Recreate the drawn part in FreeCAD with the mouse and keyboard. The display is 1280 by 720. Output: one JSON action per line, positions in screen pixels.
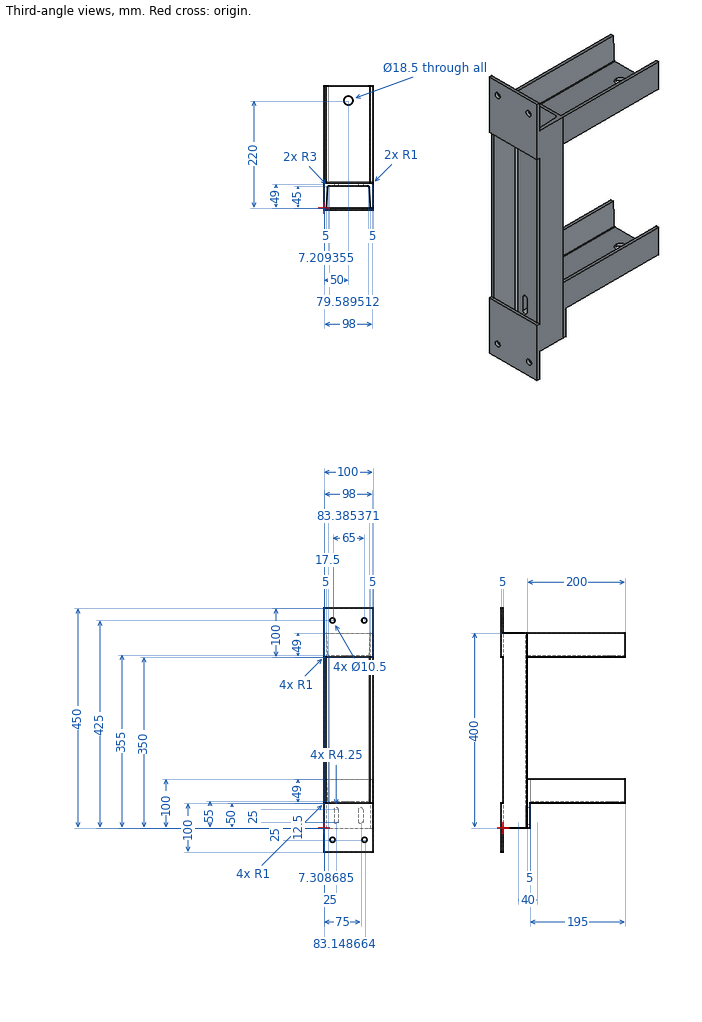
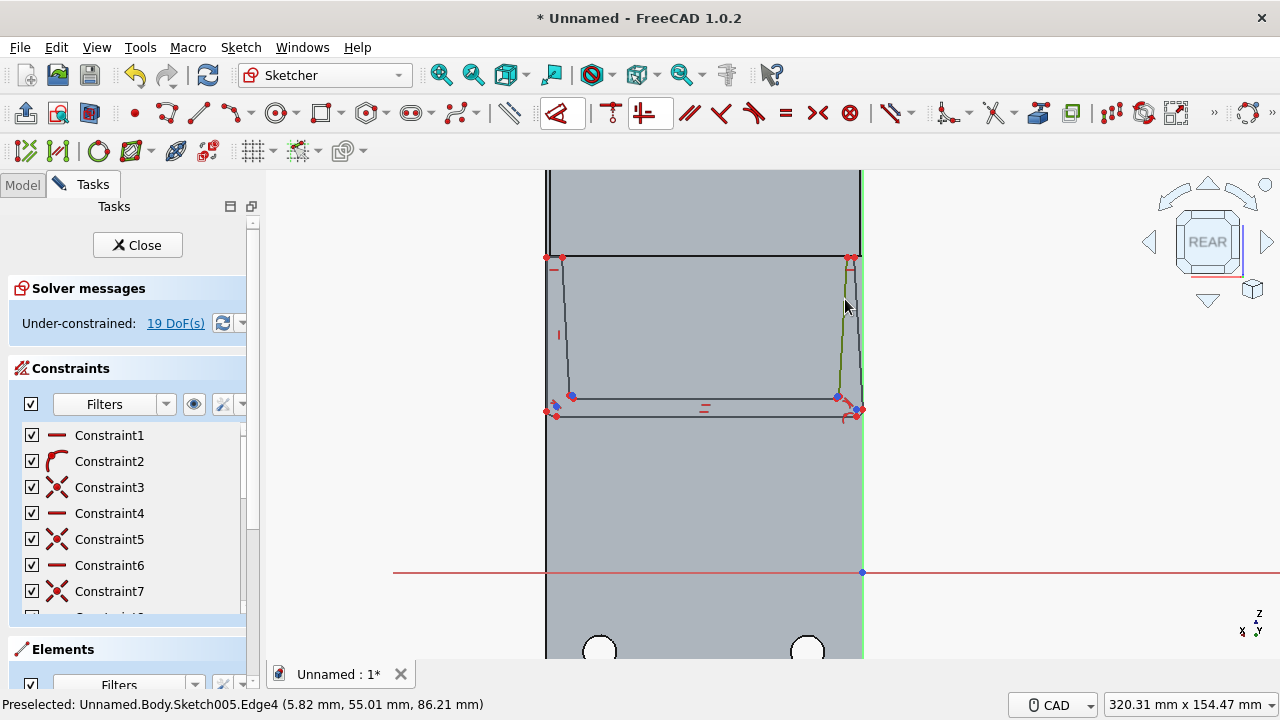
{"action": "scroll", "coordinate": [839, 398], "scroll_direction": "up", "scroll_amount": 10}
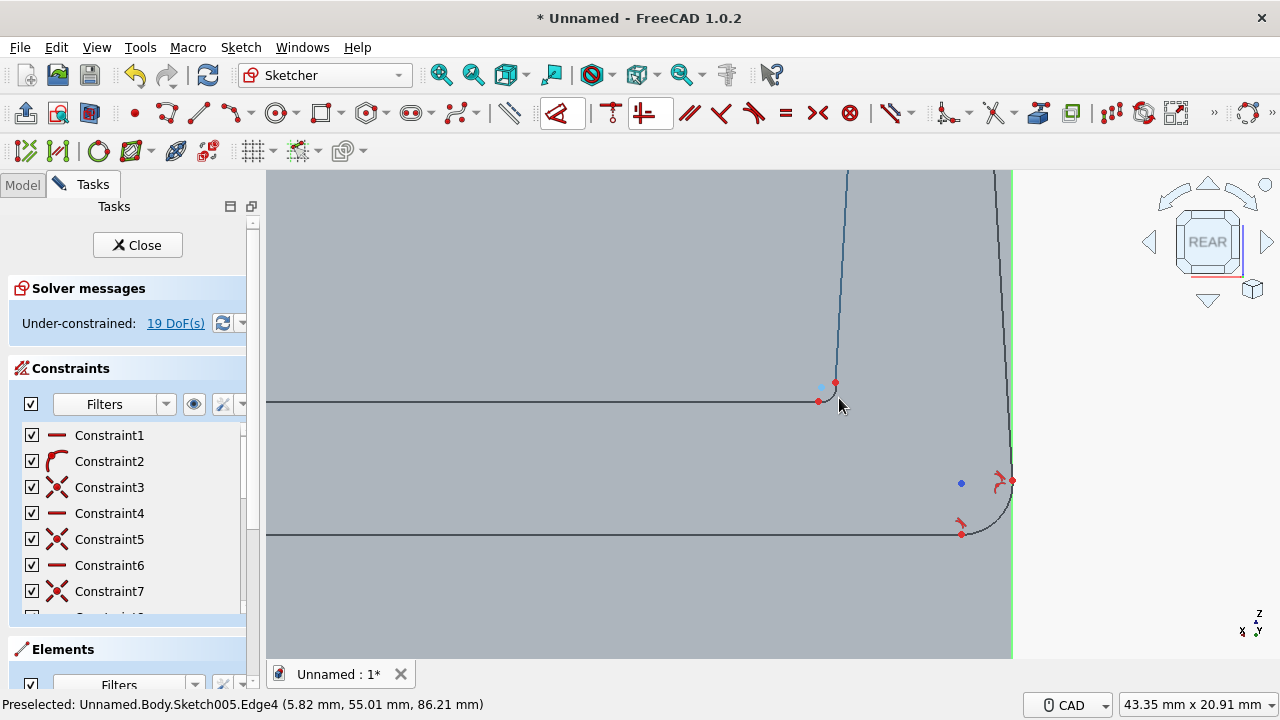
{"action": "left_click", "coordinate": [832, 397]}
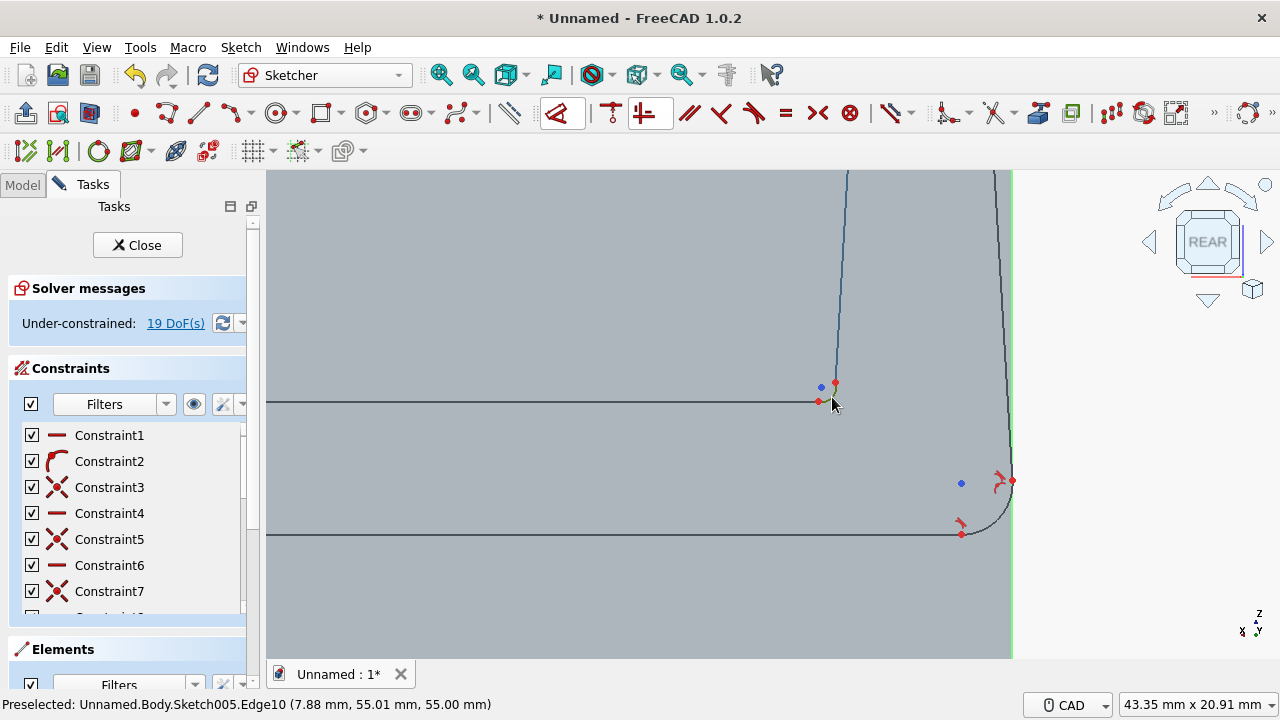
{"action": "key", "text": "t"}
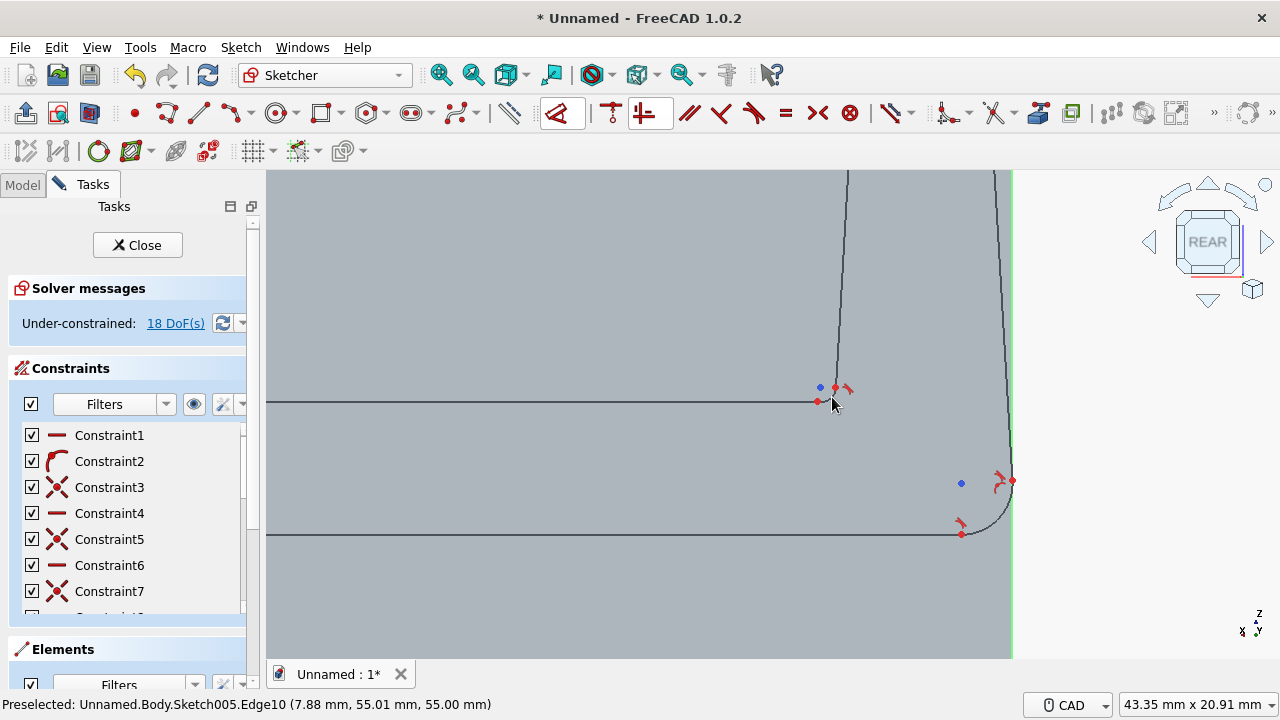
{"action": "scroll", "coordinate": [839, 398], "scroll_direction": "down", "scroll_amount": 10}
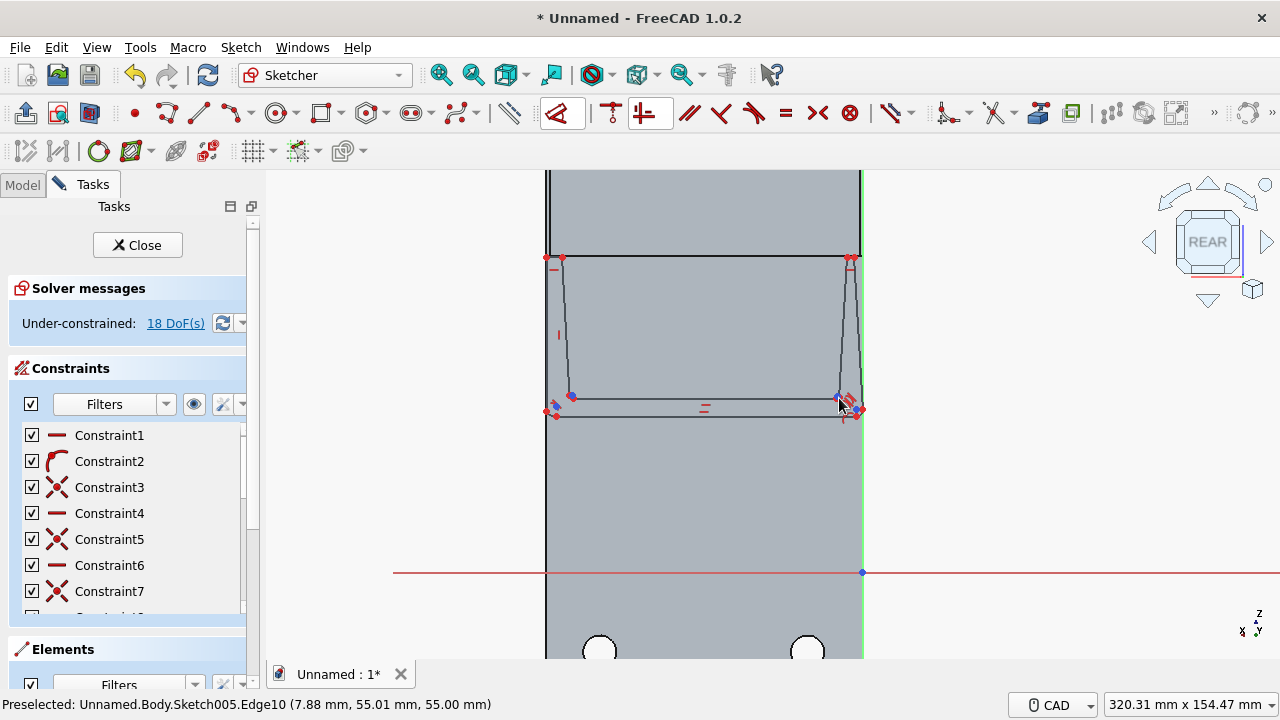
{"action": "left_click", "coordinate": [784, 399]}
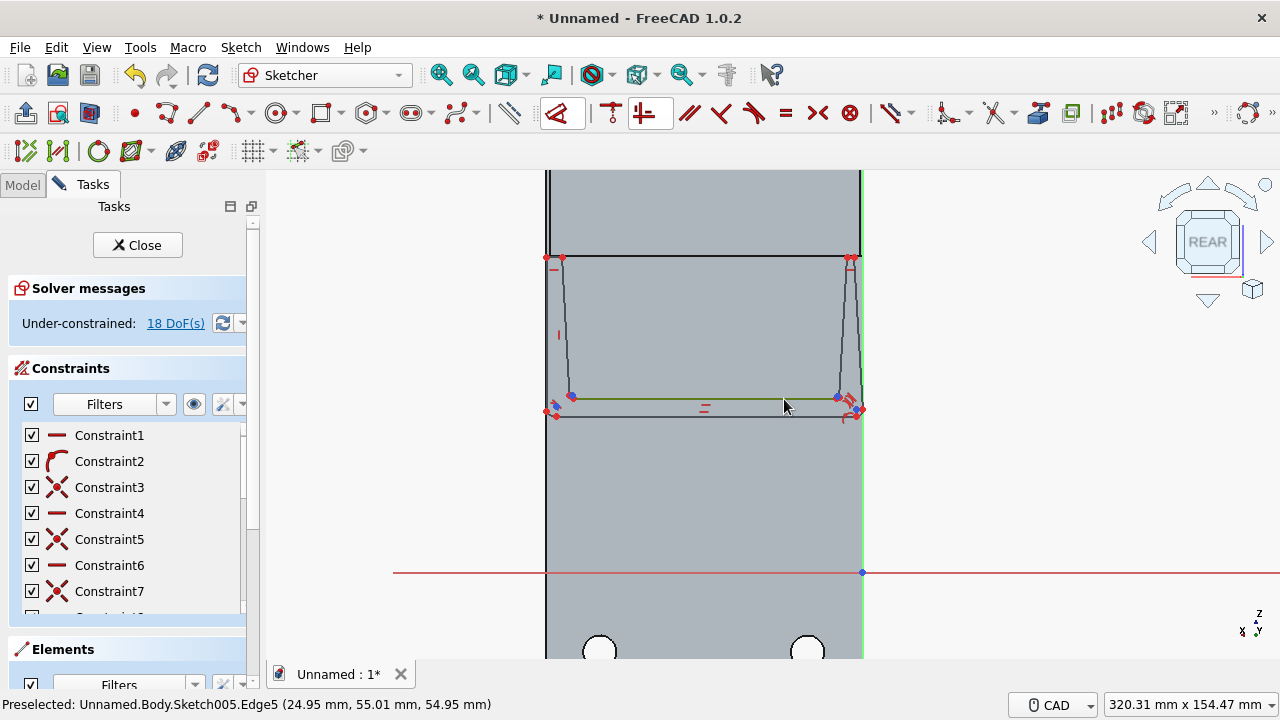
{"action": "scroll", "coordinate": [838, 399], "scroll_direction": "up", "scroll_amount": 11}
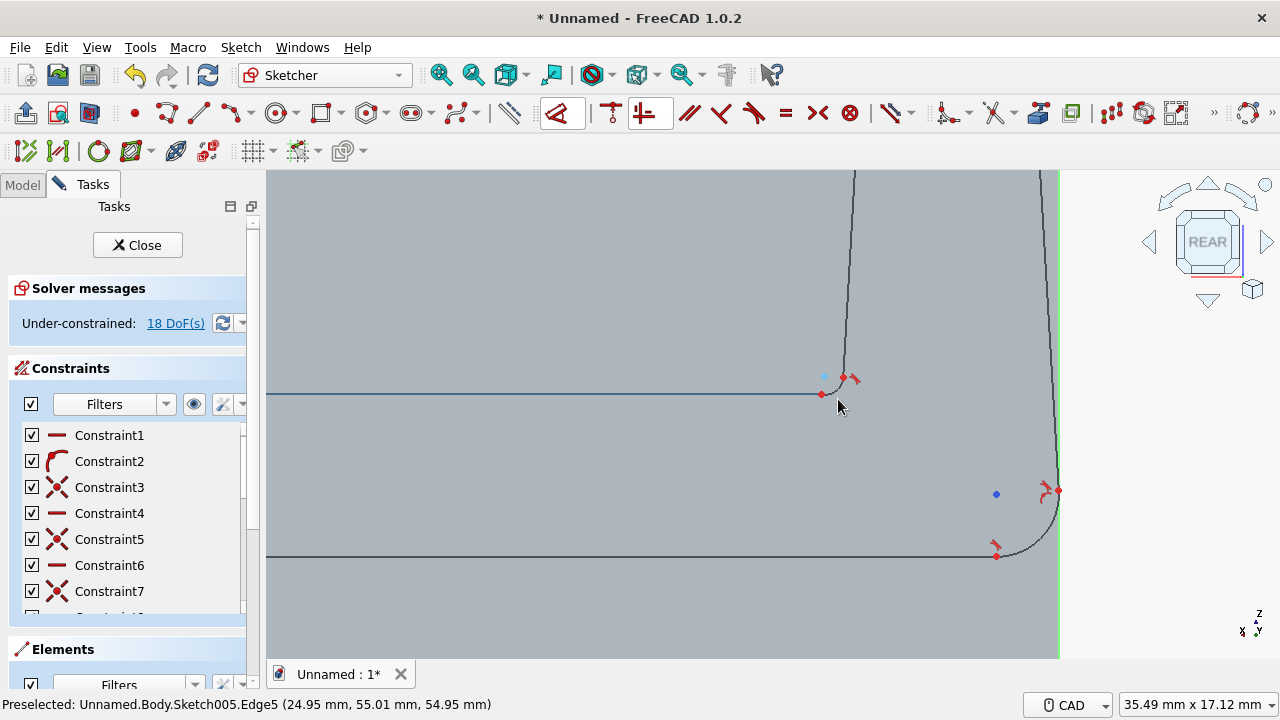
{"action": "left_click", "coordinate": [836, 391]}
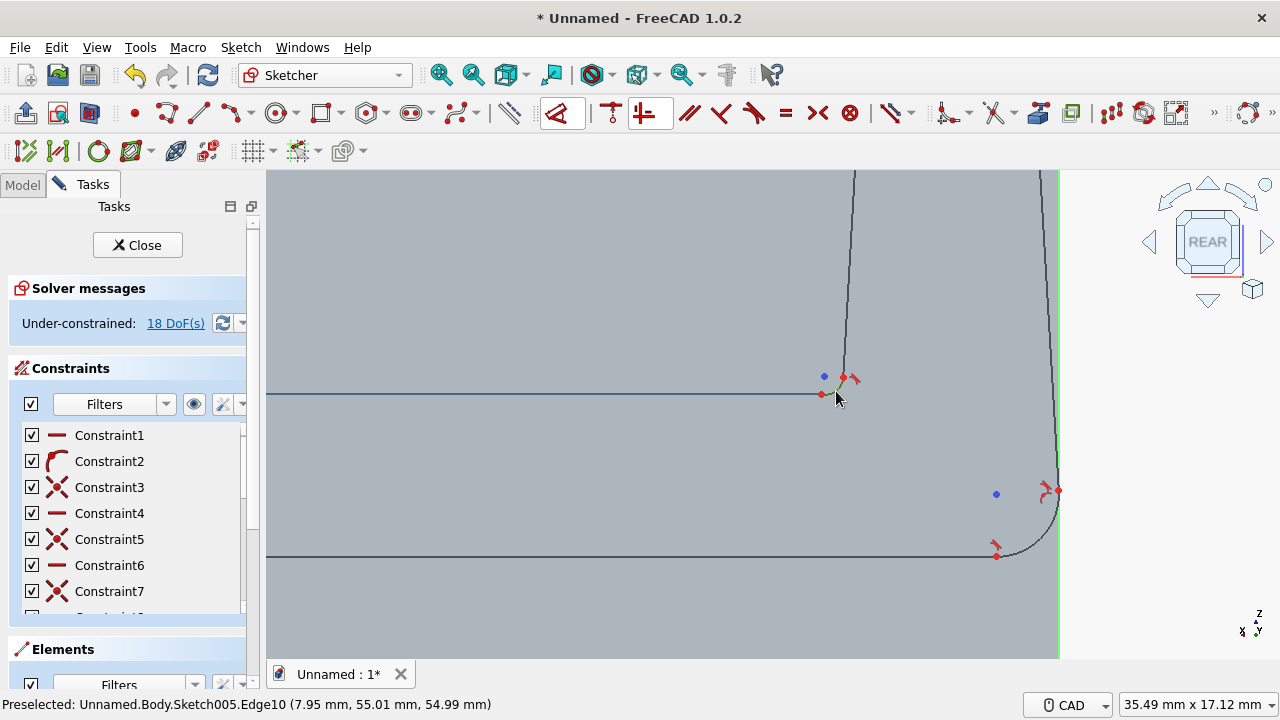
{"action": "left_click", "coordinate": [754, 114]}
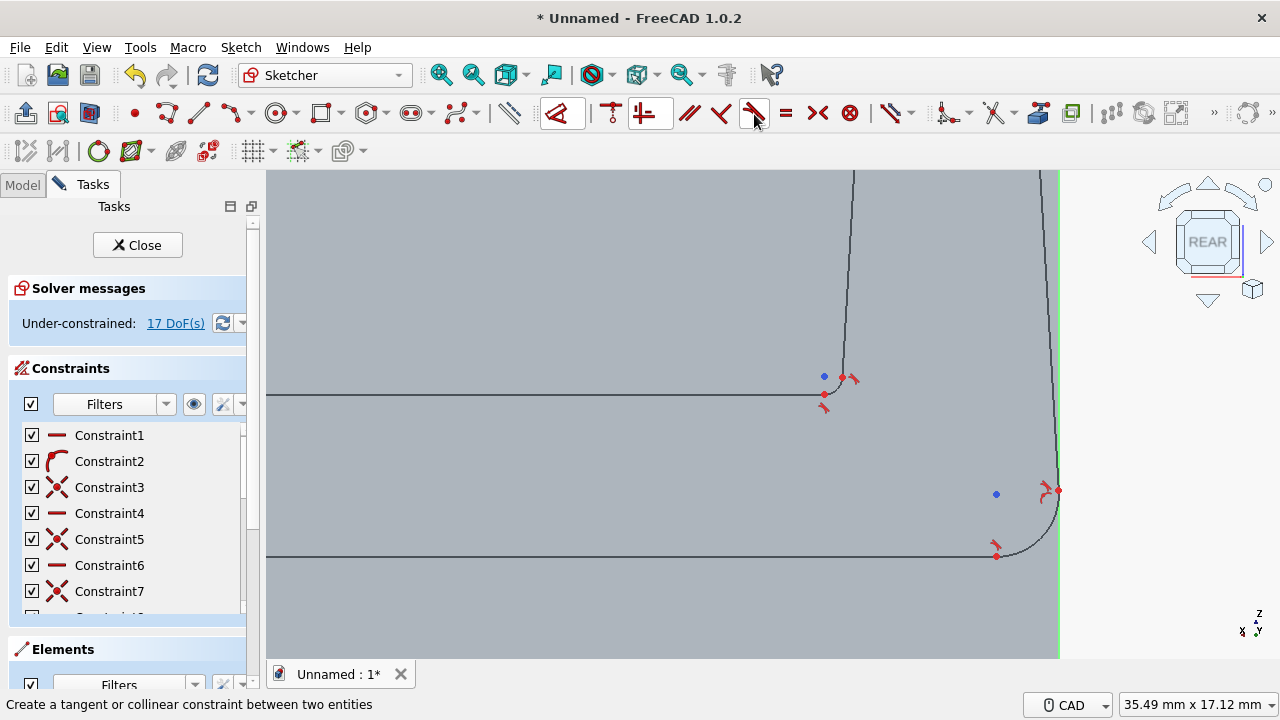
{"action": "scroll", "coordinate": [838, 399], "scroll_direction": "down", "scroll_amount": 11}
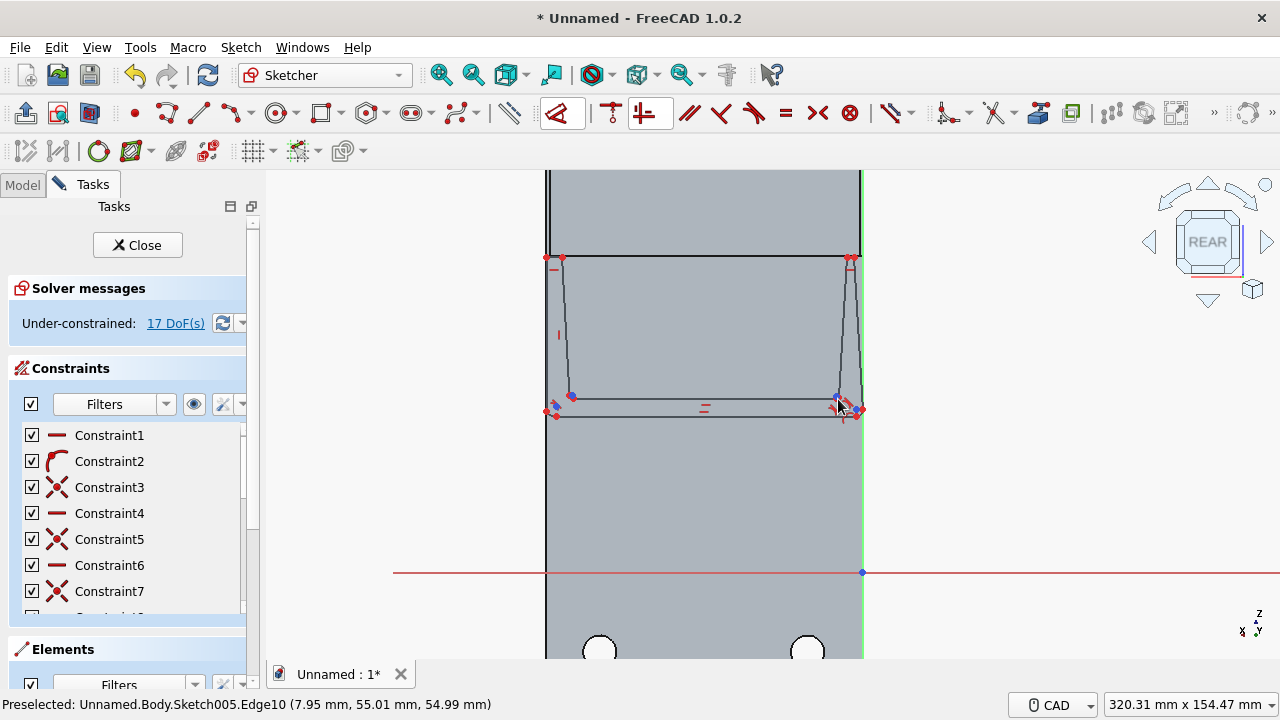
{"action": "left_click", "coordinate": [784, 399]}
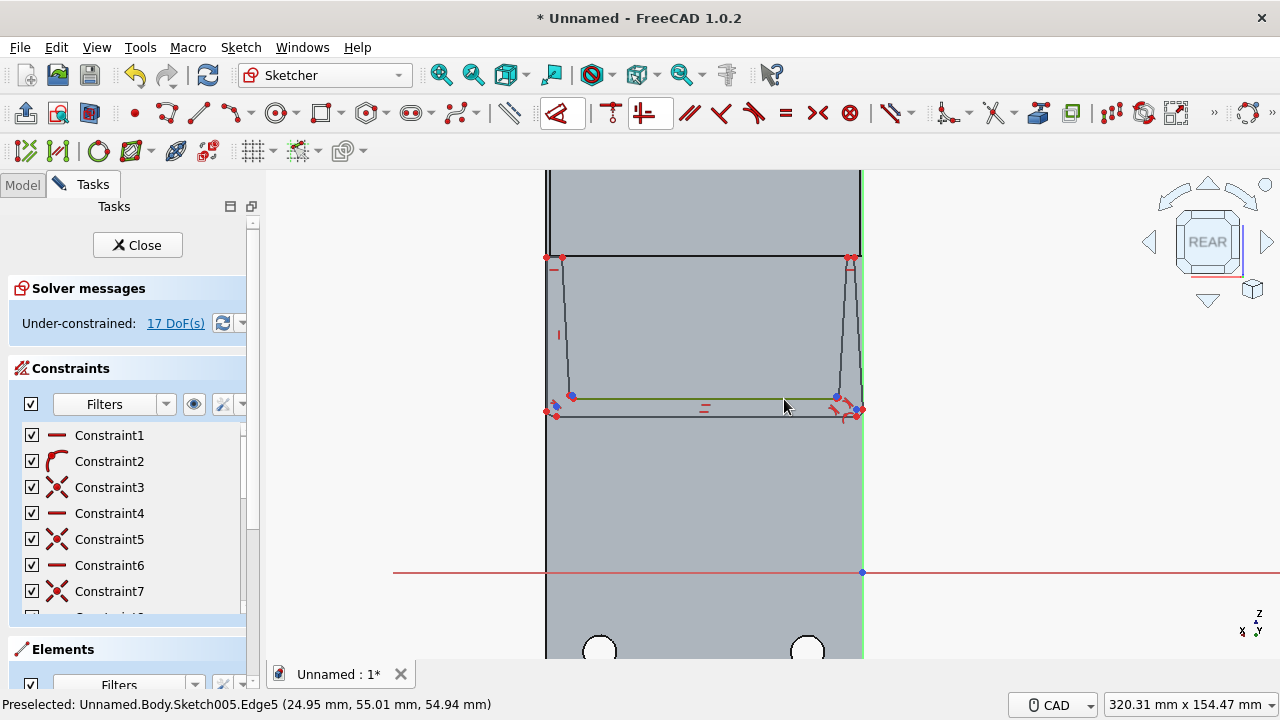
{"action": "scroll", "coordinate": [571, 398], "scroll_direction": "up", "scroll_amount": 9}